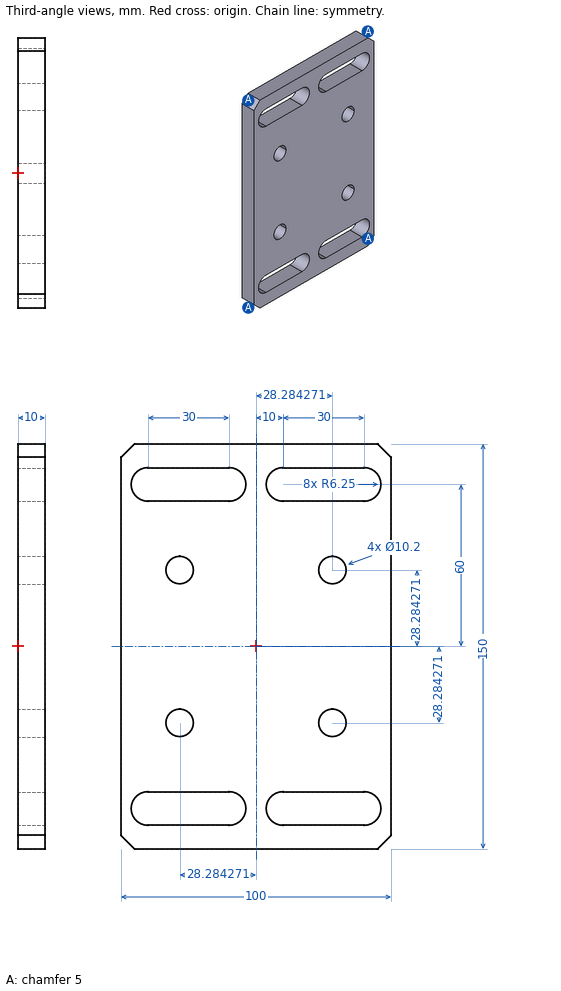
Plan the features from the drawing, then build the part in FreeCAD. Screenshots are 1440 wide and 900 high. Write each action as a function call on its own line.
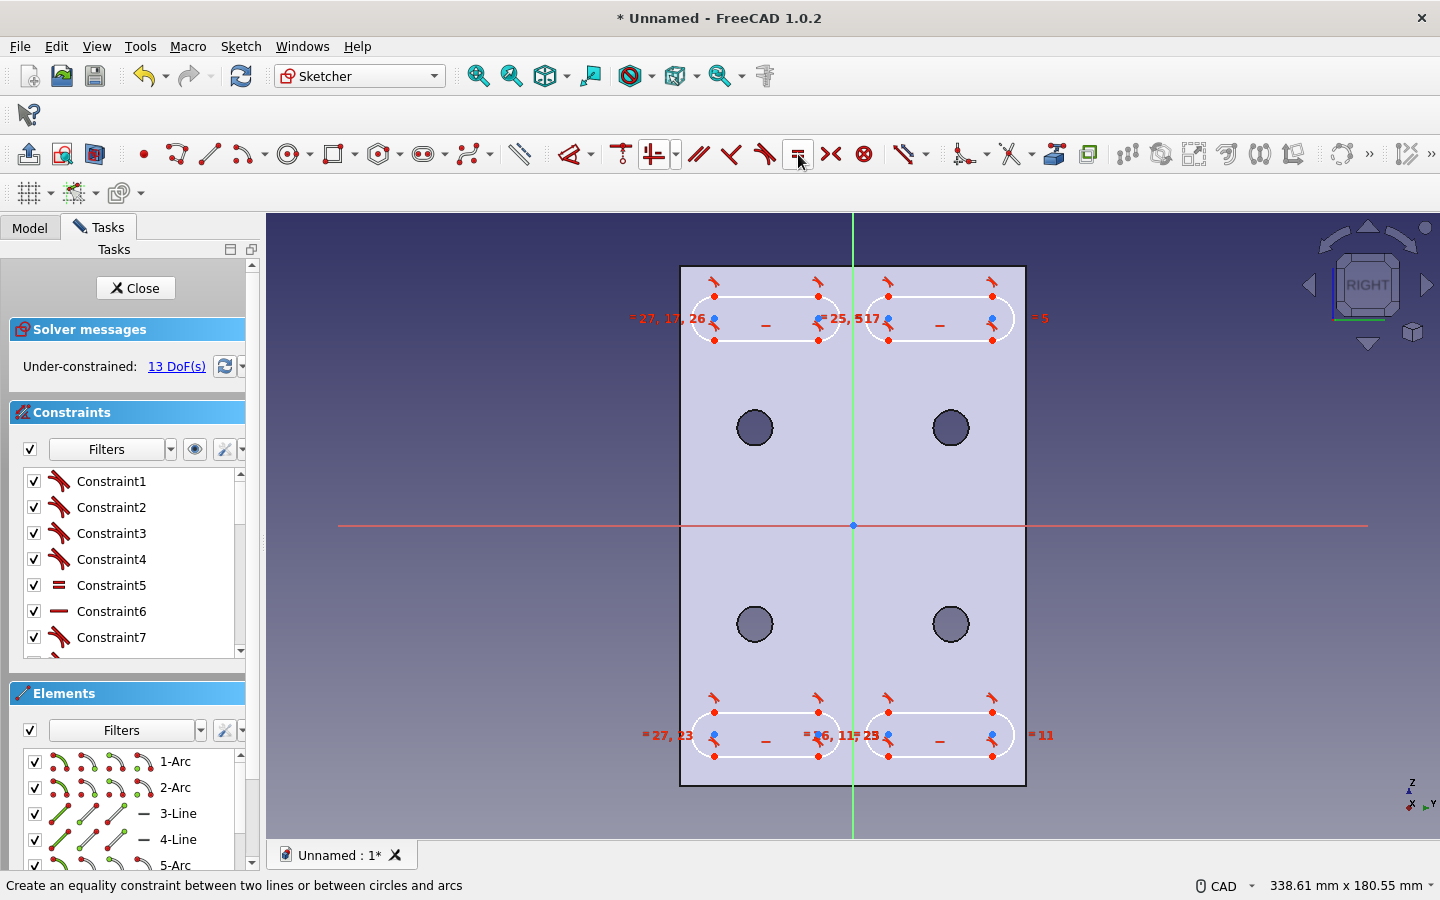
click(888, 319)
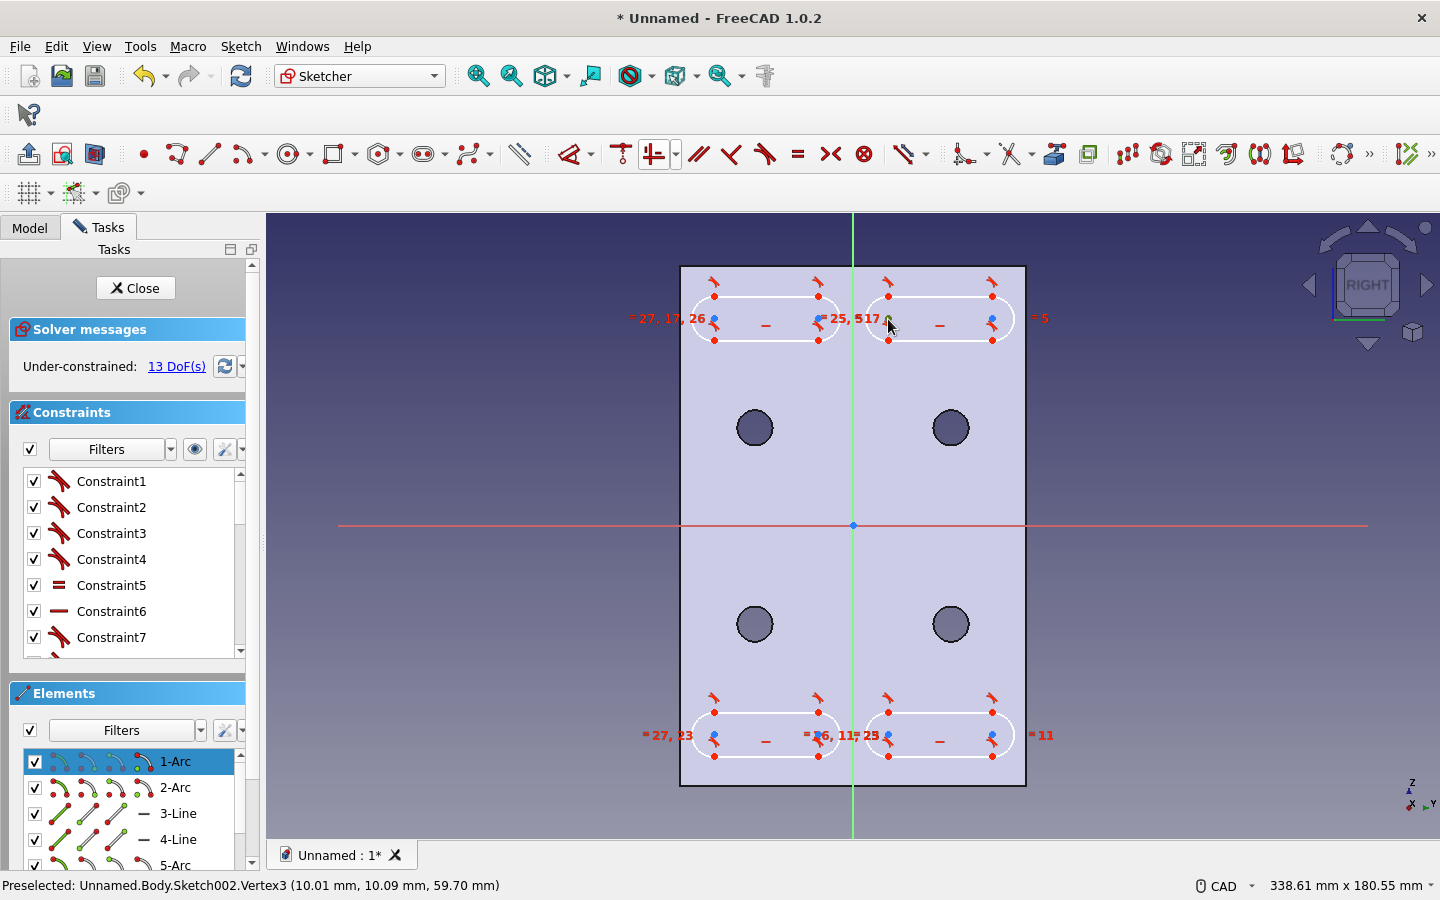
click(888, 735)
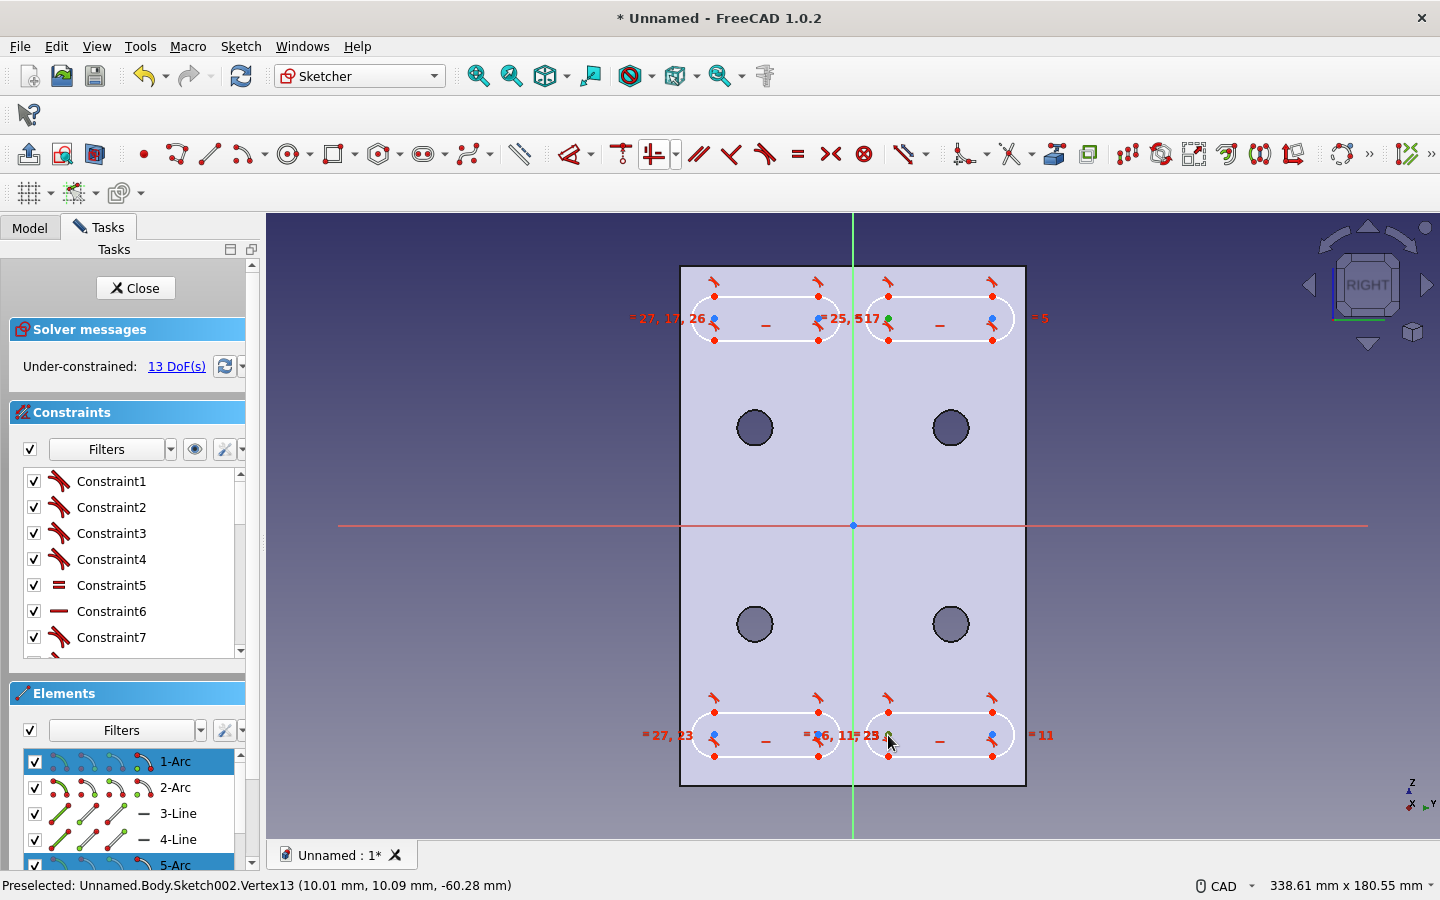
click(364, 526)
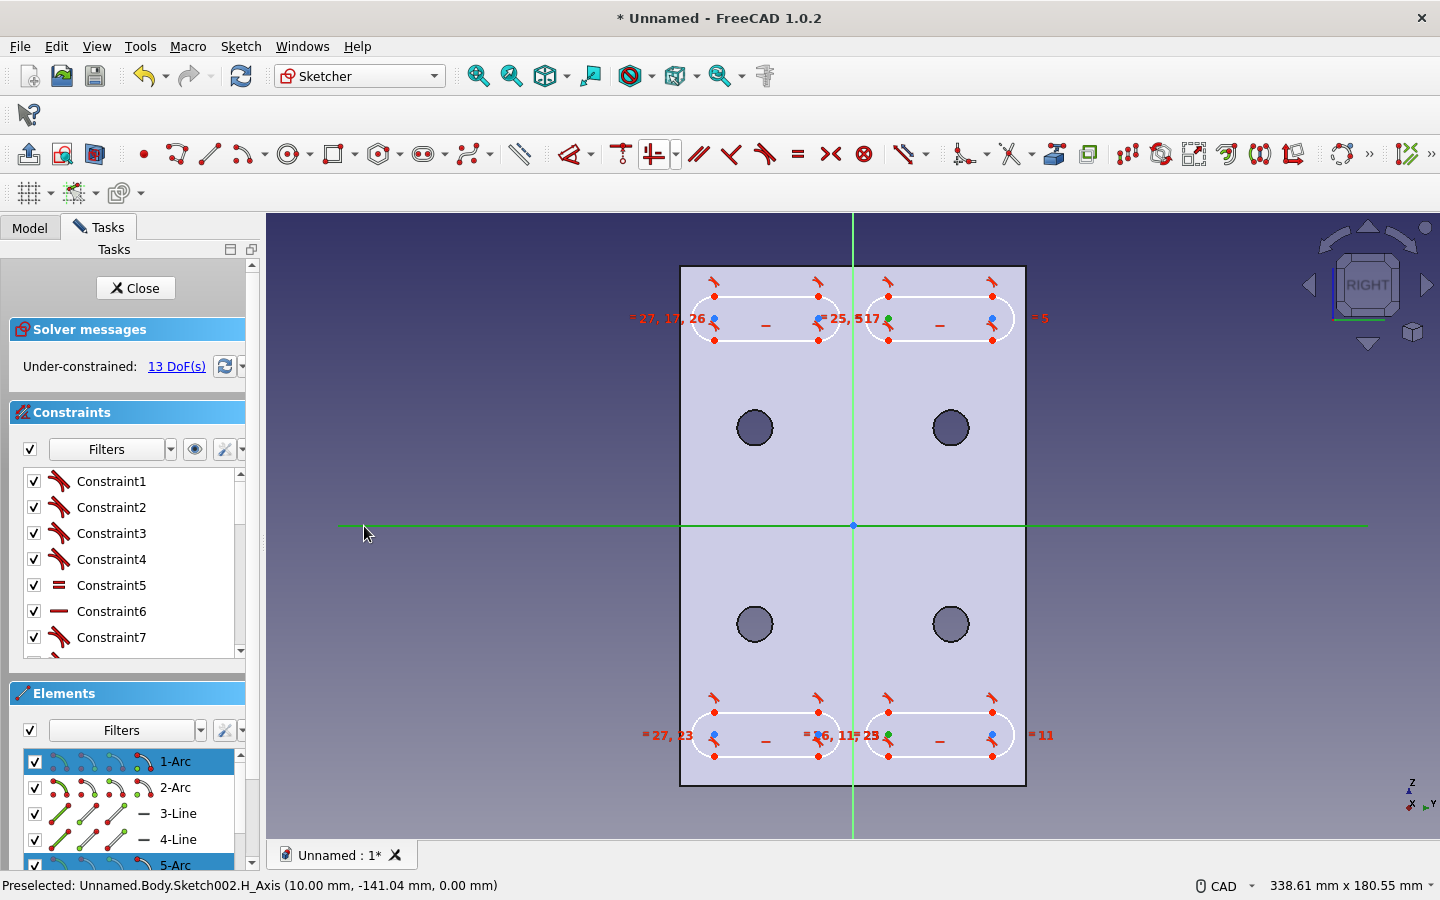
click(831, 154)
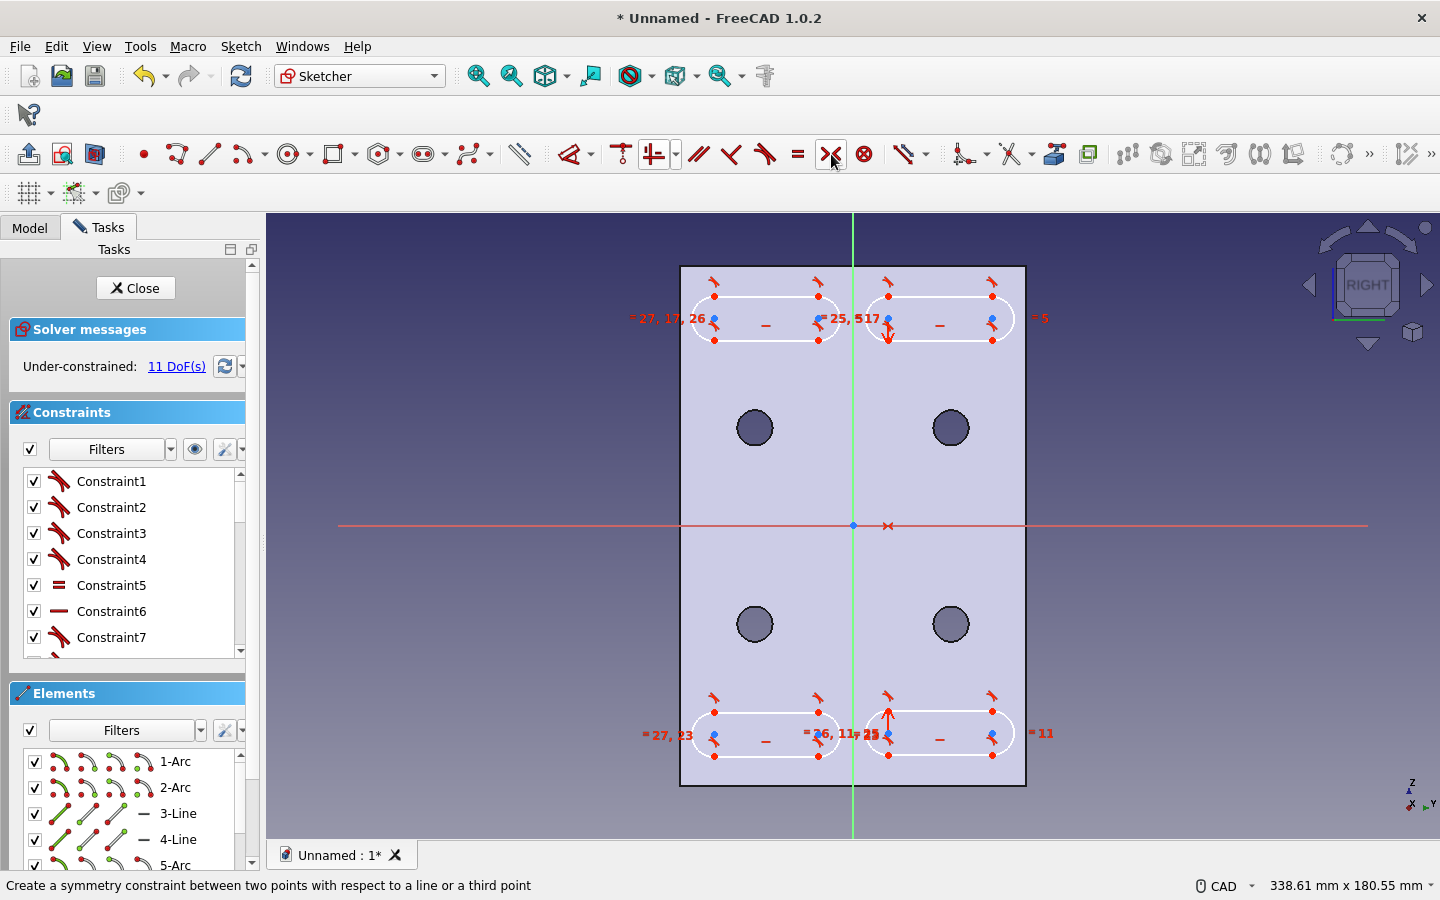
click(992, 319)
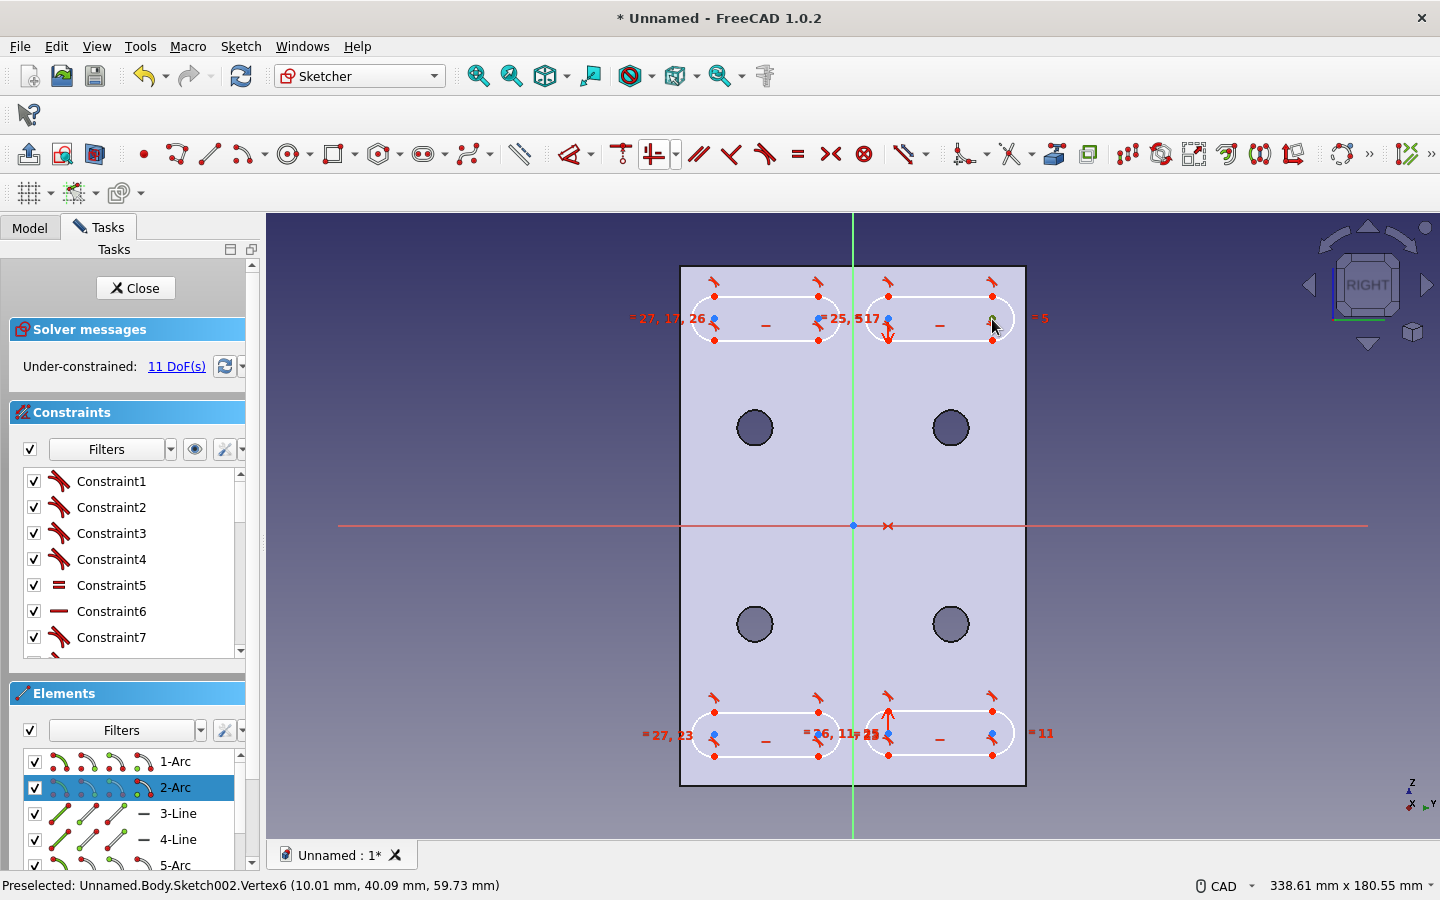
click(714, 319)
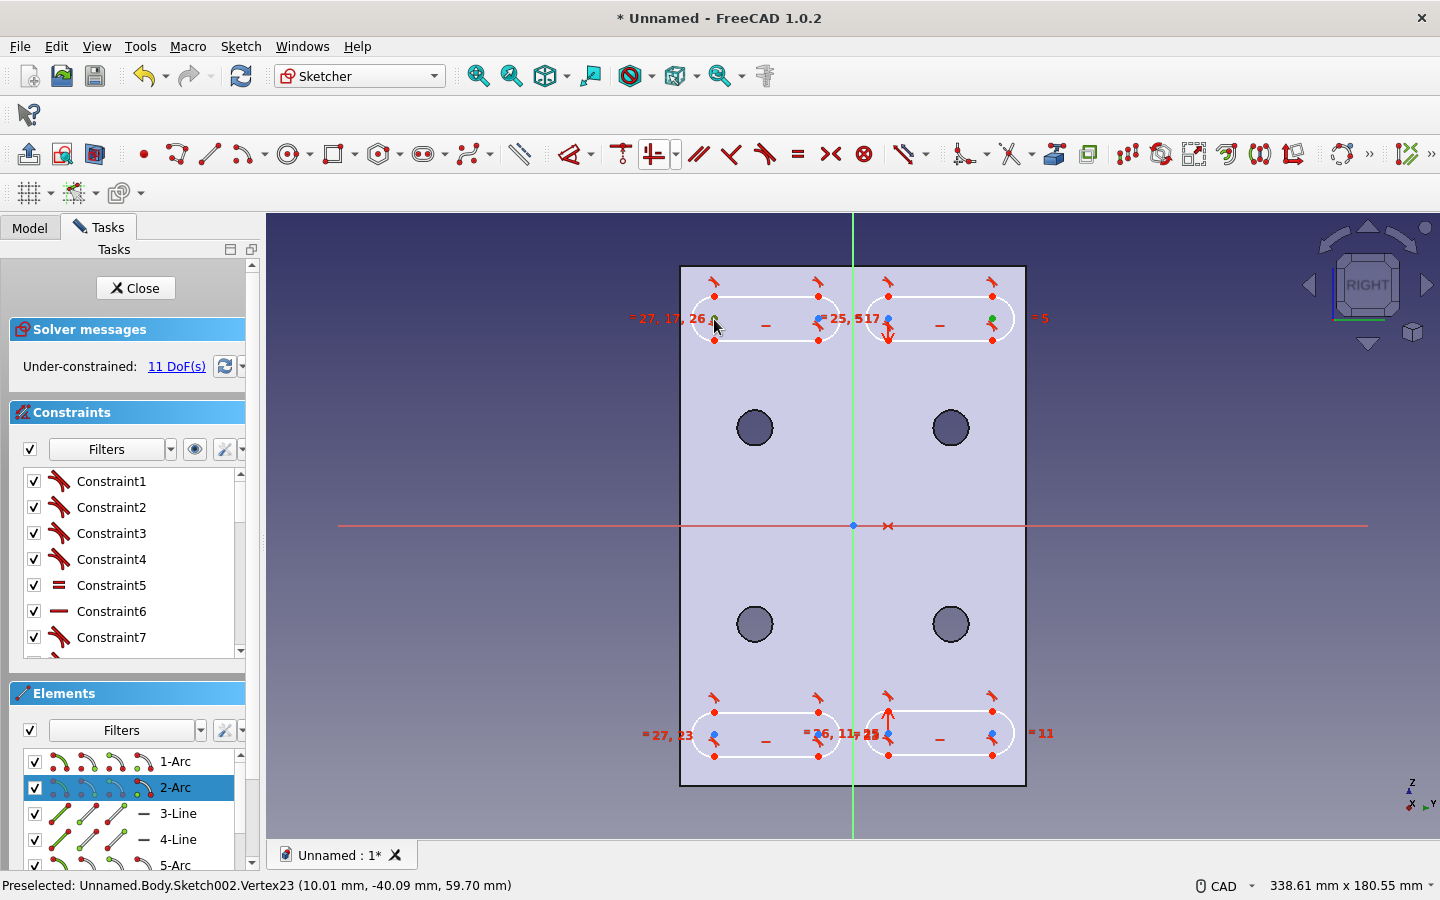
click(853, 689)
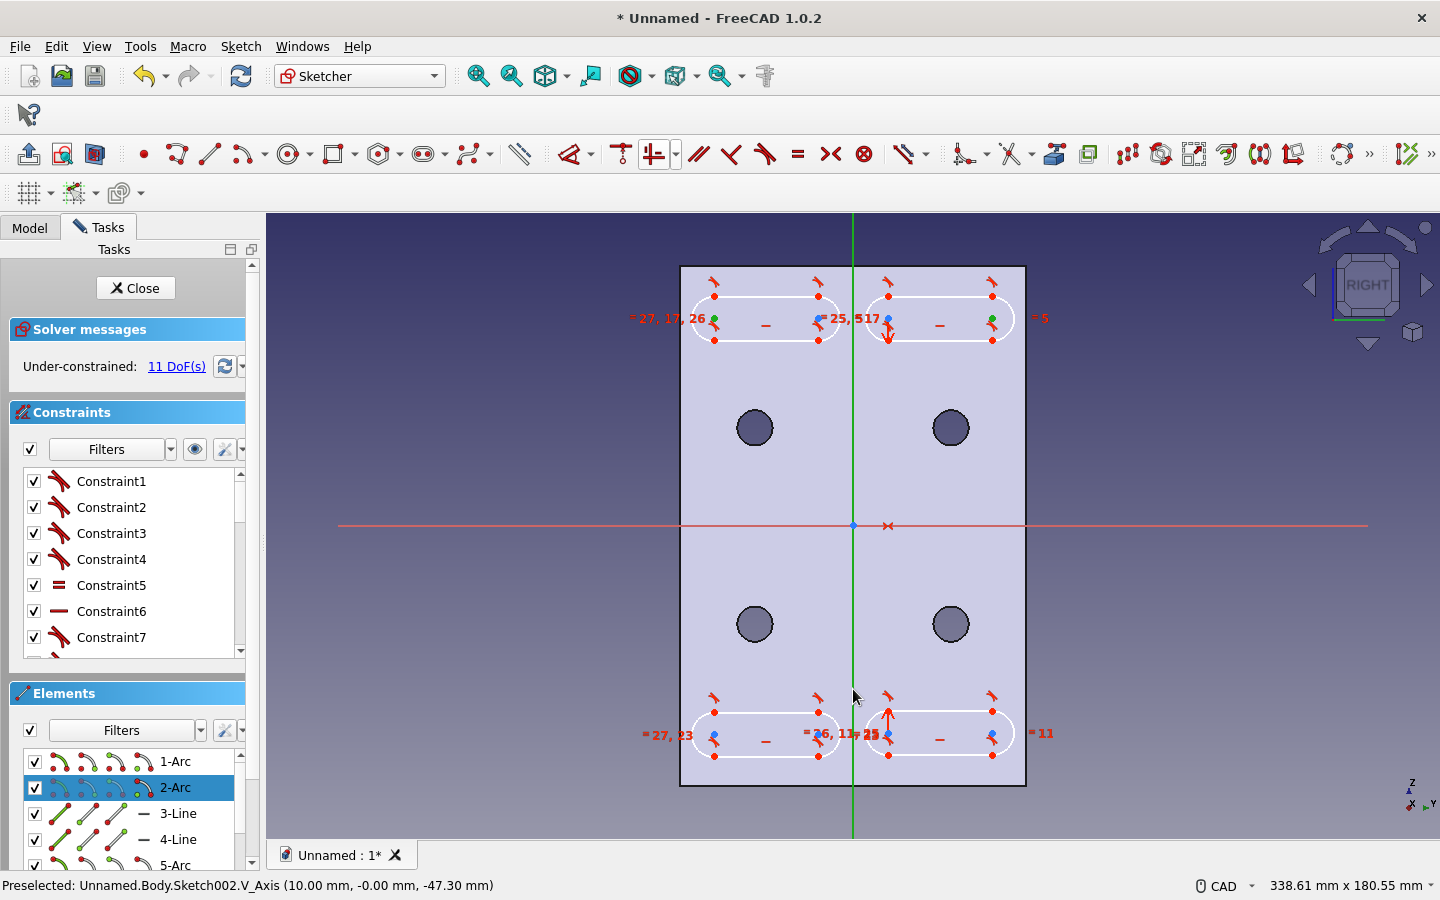
key(s)